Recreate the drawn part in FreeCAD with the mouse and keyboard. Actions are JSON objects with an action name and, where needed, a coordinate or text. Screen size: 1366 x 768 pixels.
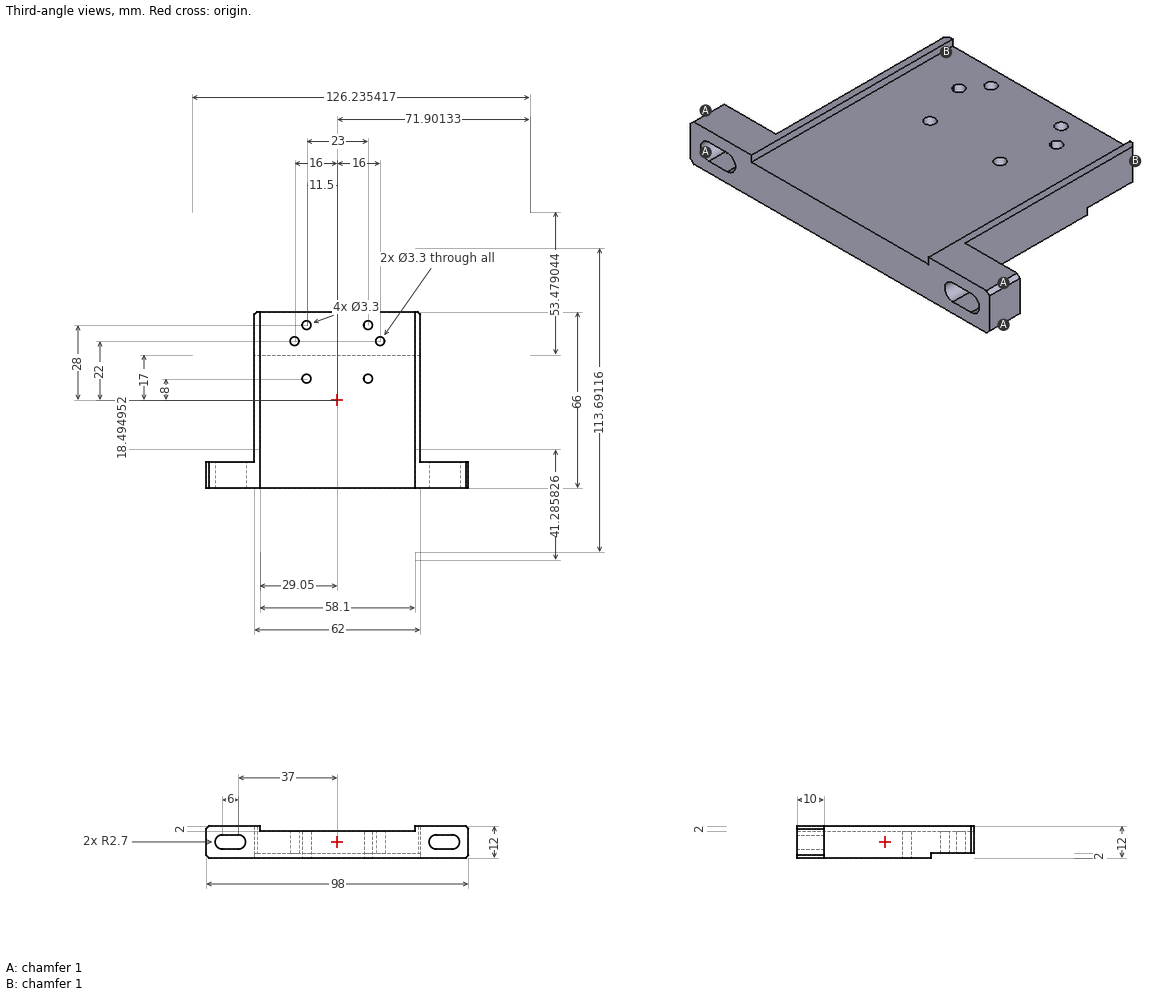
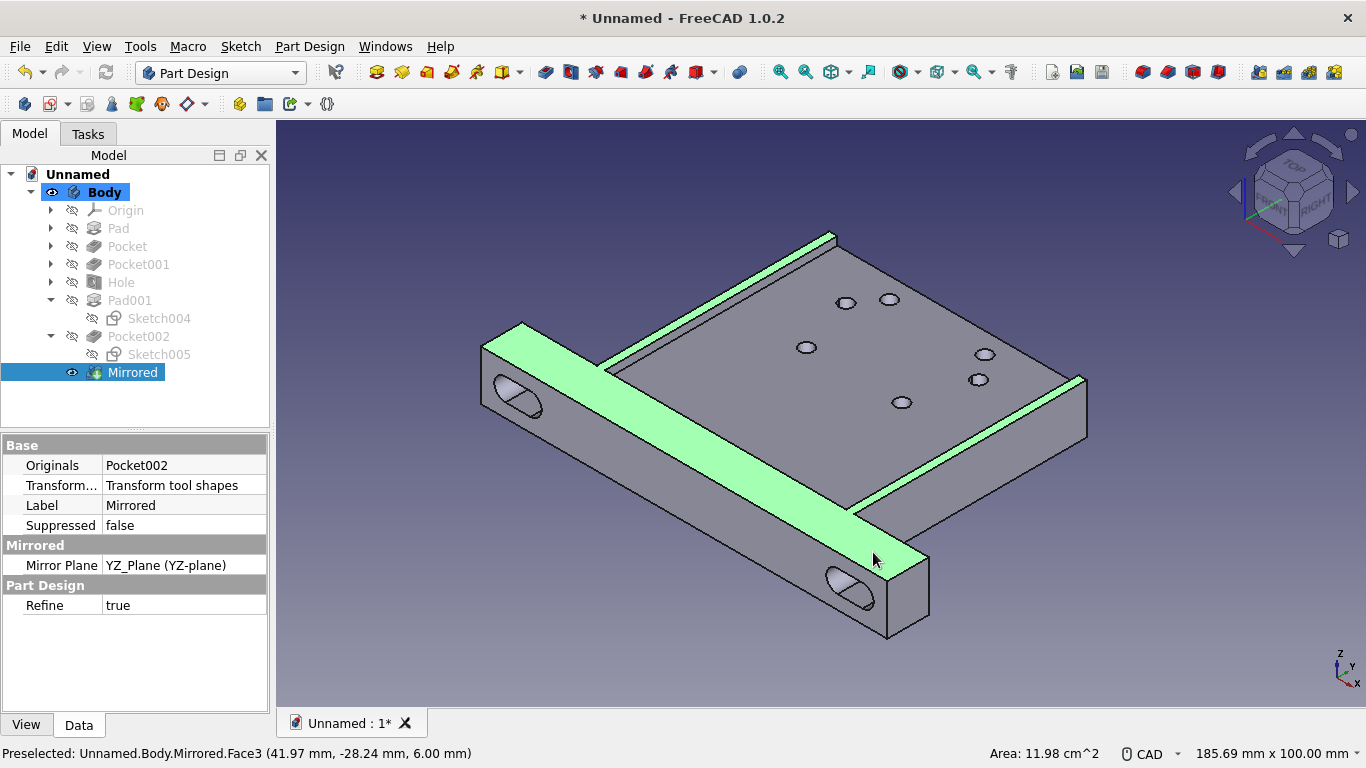
{"action": "left_click", "coordinate": [50, 104]}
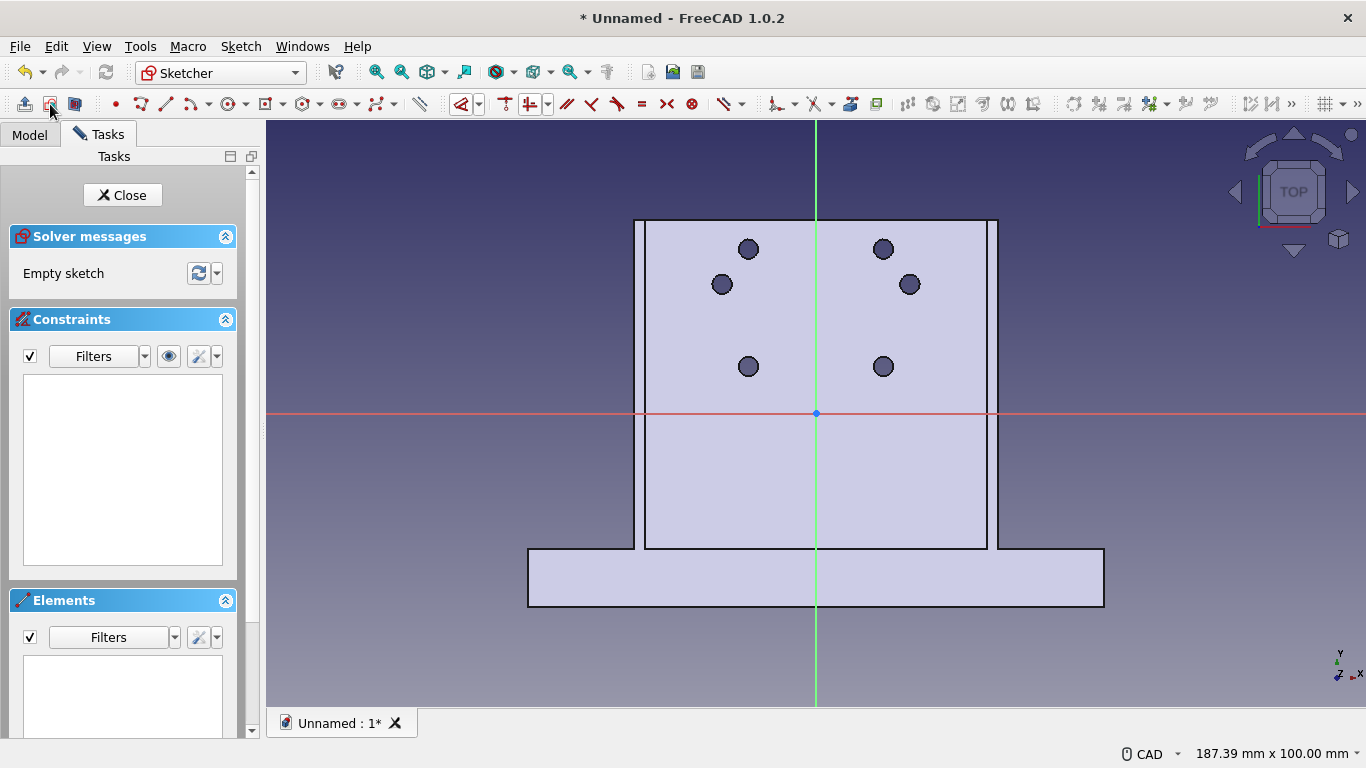
{"action": "scroll", "coordinate": [438, 148], "scroll_direction": "down", "scroll_amount": 1}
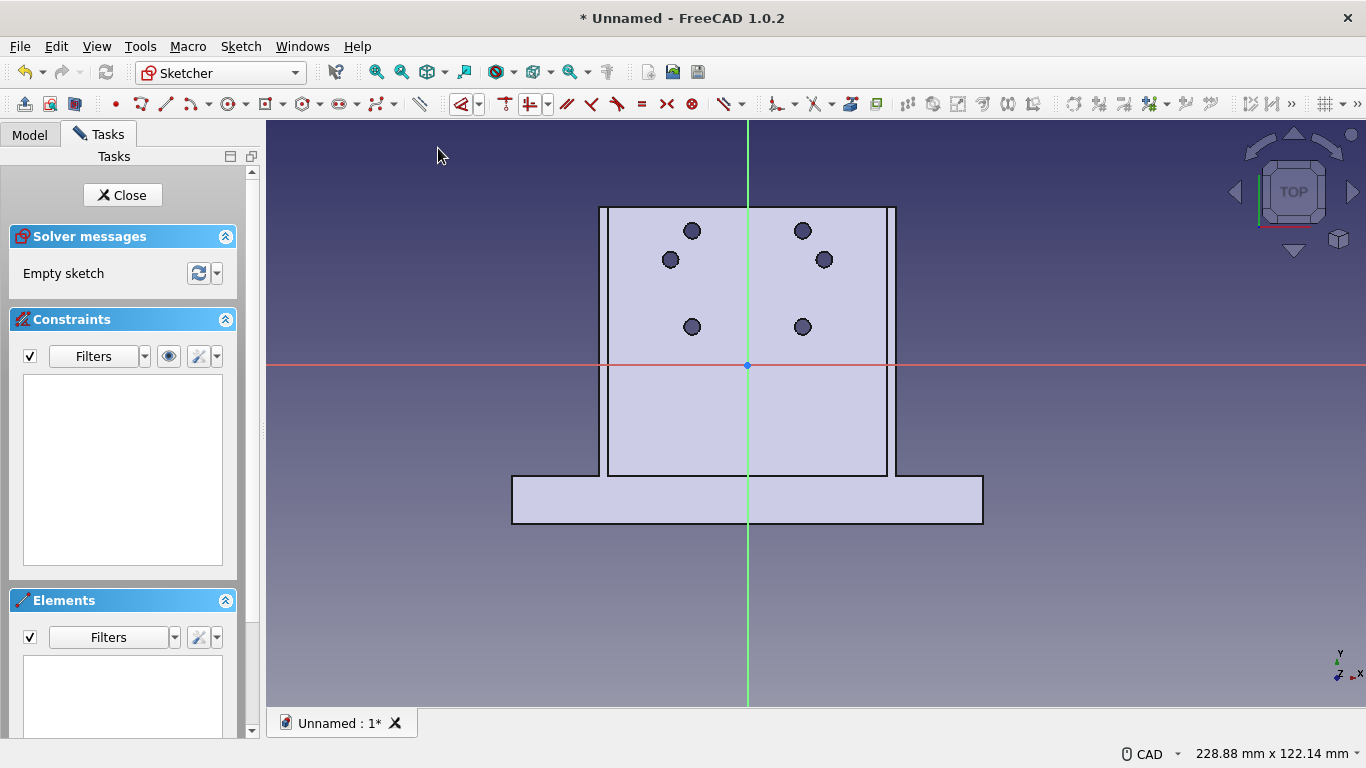
{"action": "left_click", "coordinate": [282, 104]}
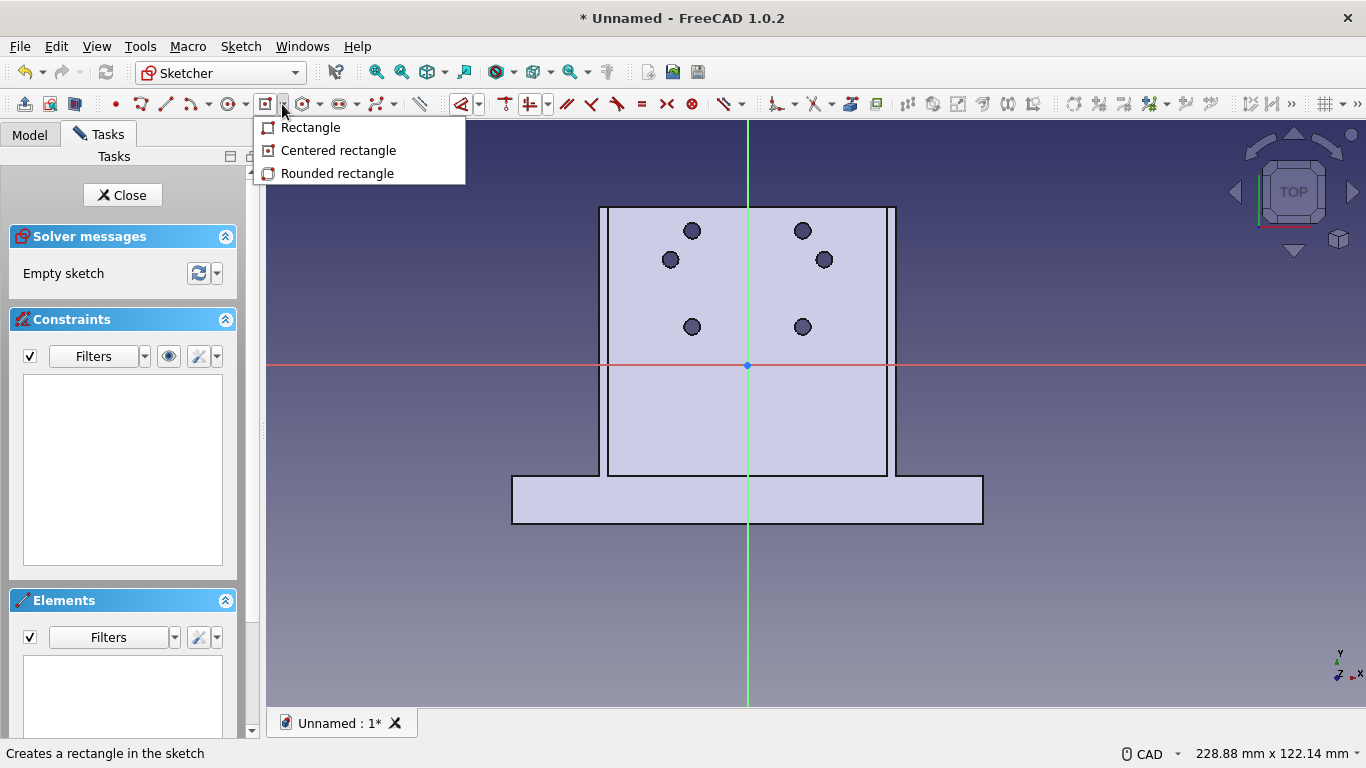
{"action": "left_click", "coordinate": [360, 128]}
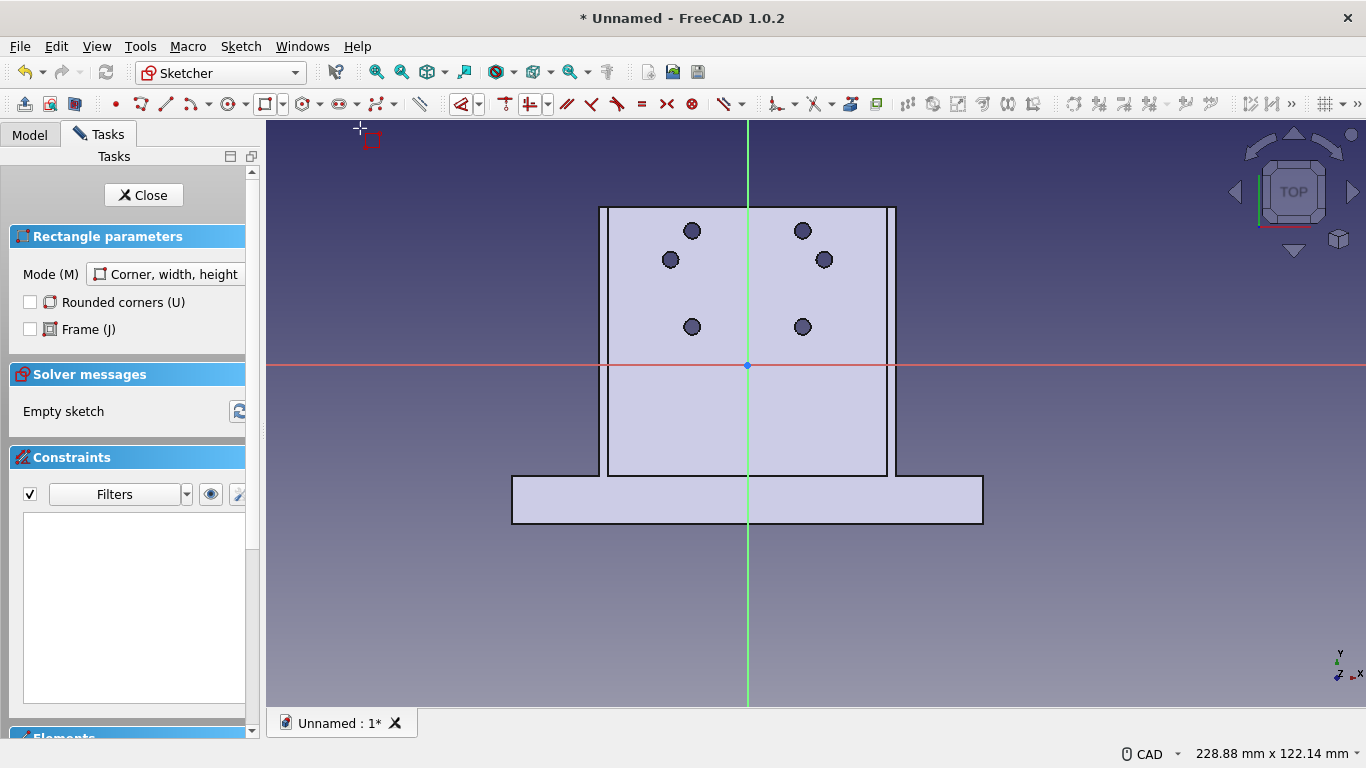
{"action": "left_click", "coordinate": [608, 454]}
{"action": "mouse_move", "coordinate": [887, 653]}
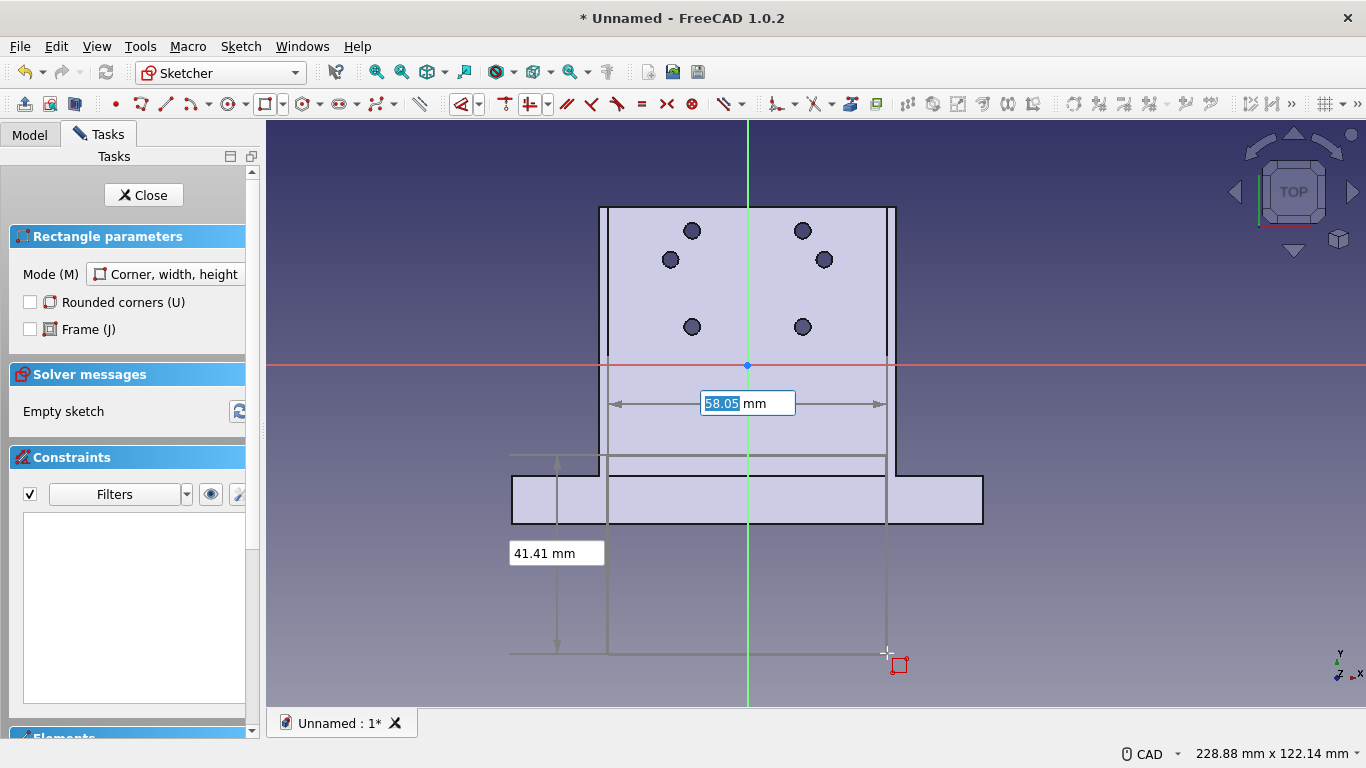
{"action": "type", "text": "58.1"}
{"action": "key", "text": "Tab"}
{"action": "type", "text": "41.285826"}
{"action": "key", "text": "Return"}
{"action": "key", "text": "Escape"}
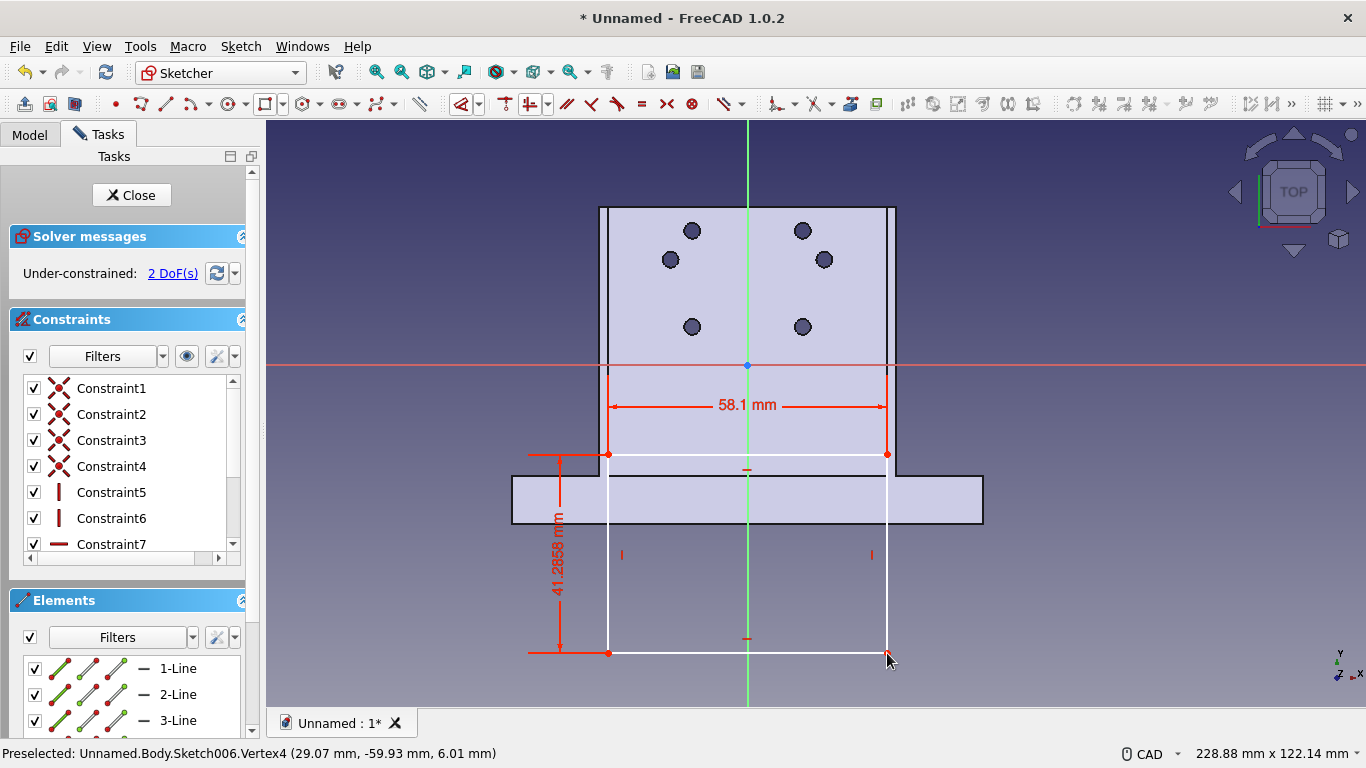
{"action": "left_click", "coordinate": [608, 455]}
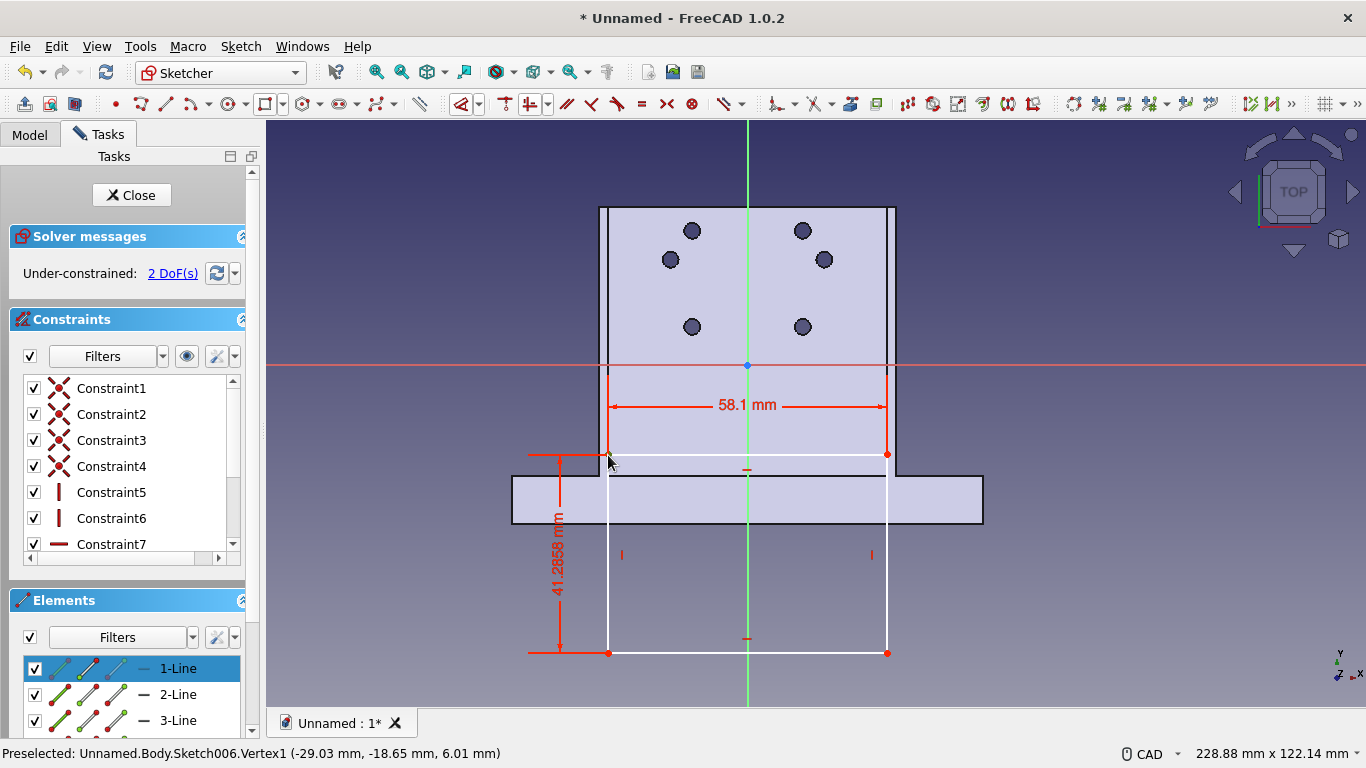
{"action": "key", "text": "l"}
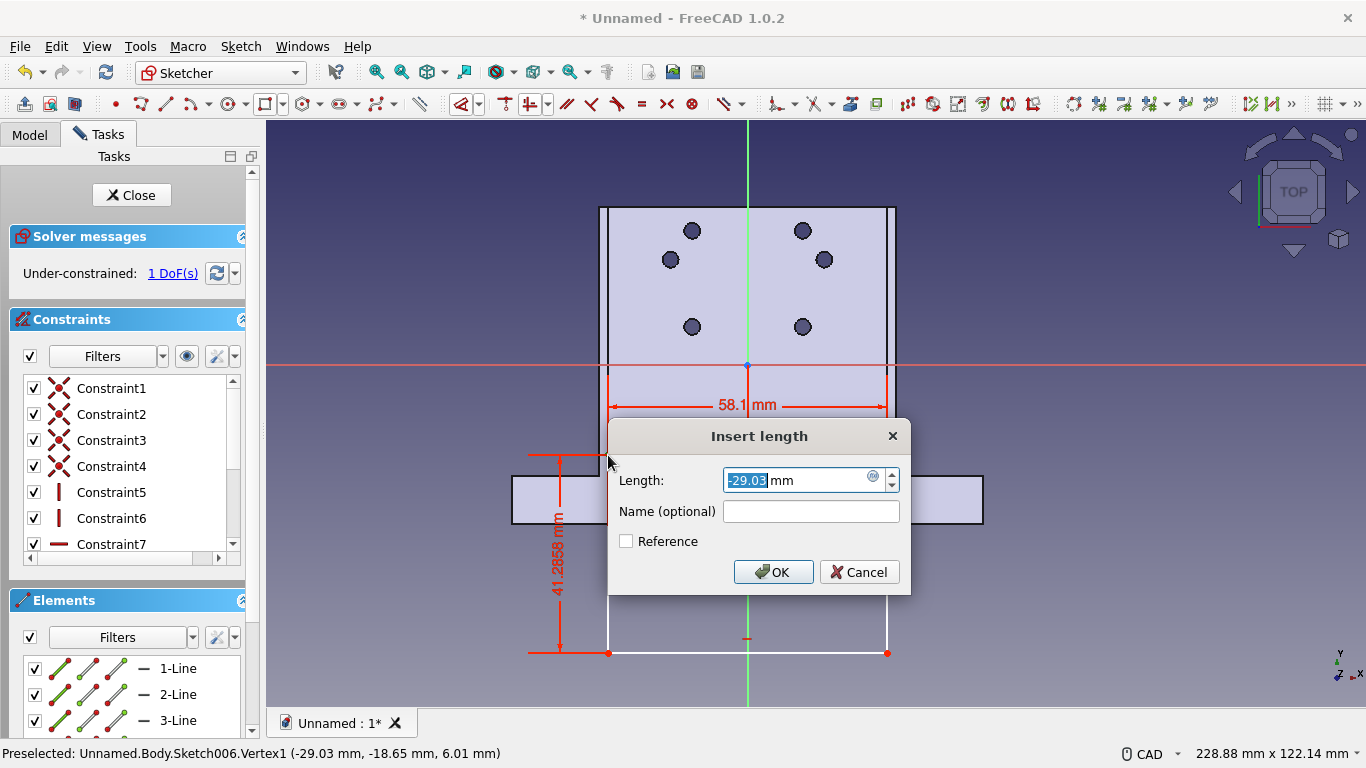
{"action": "type", "text": "-29.05"}
{"action": "key", "text": "Return"}